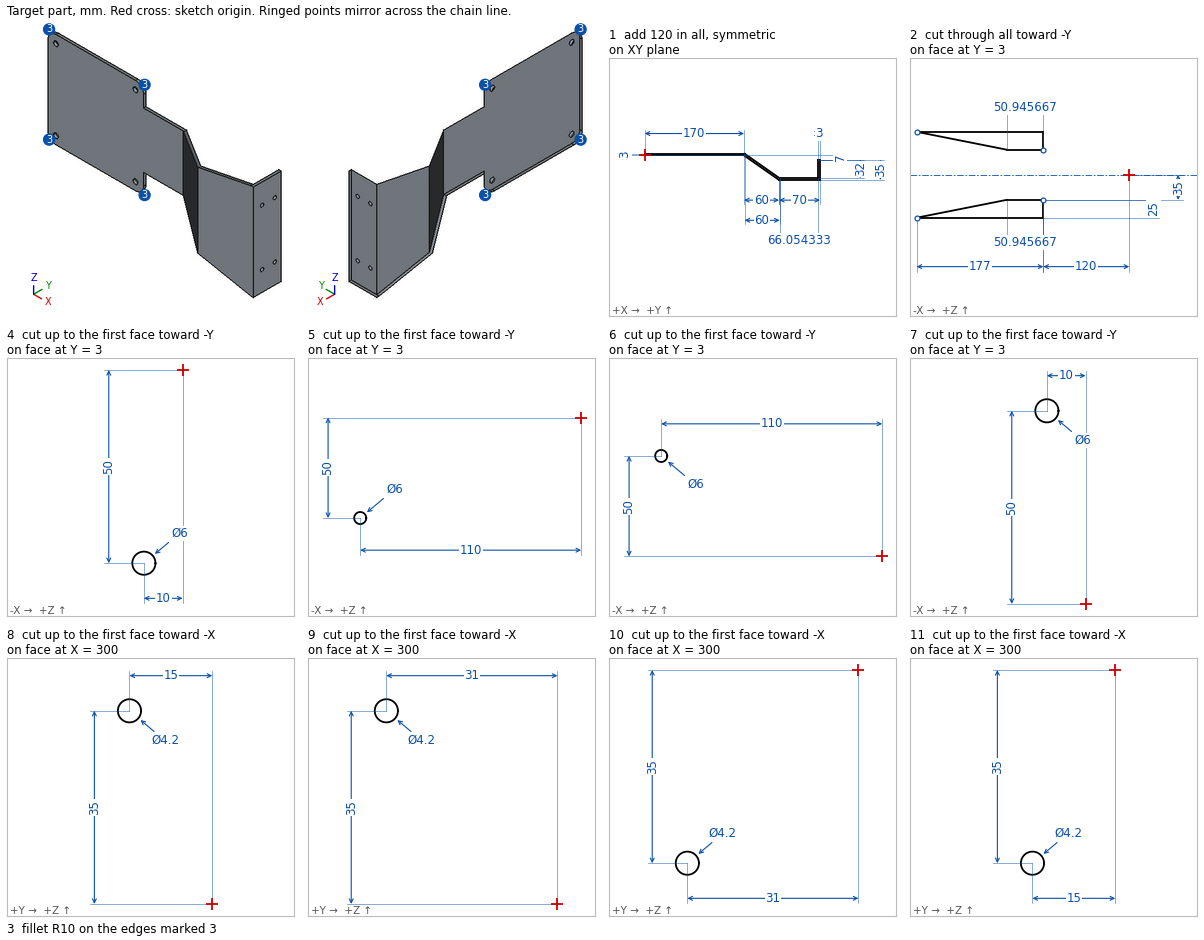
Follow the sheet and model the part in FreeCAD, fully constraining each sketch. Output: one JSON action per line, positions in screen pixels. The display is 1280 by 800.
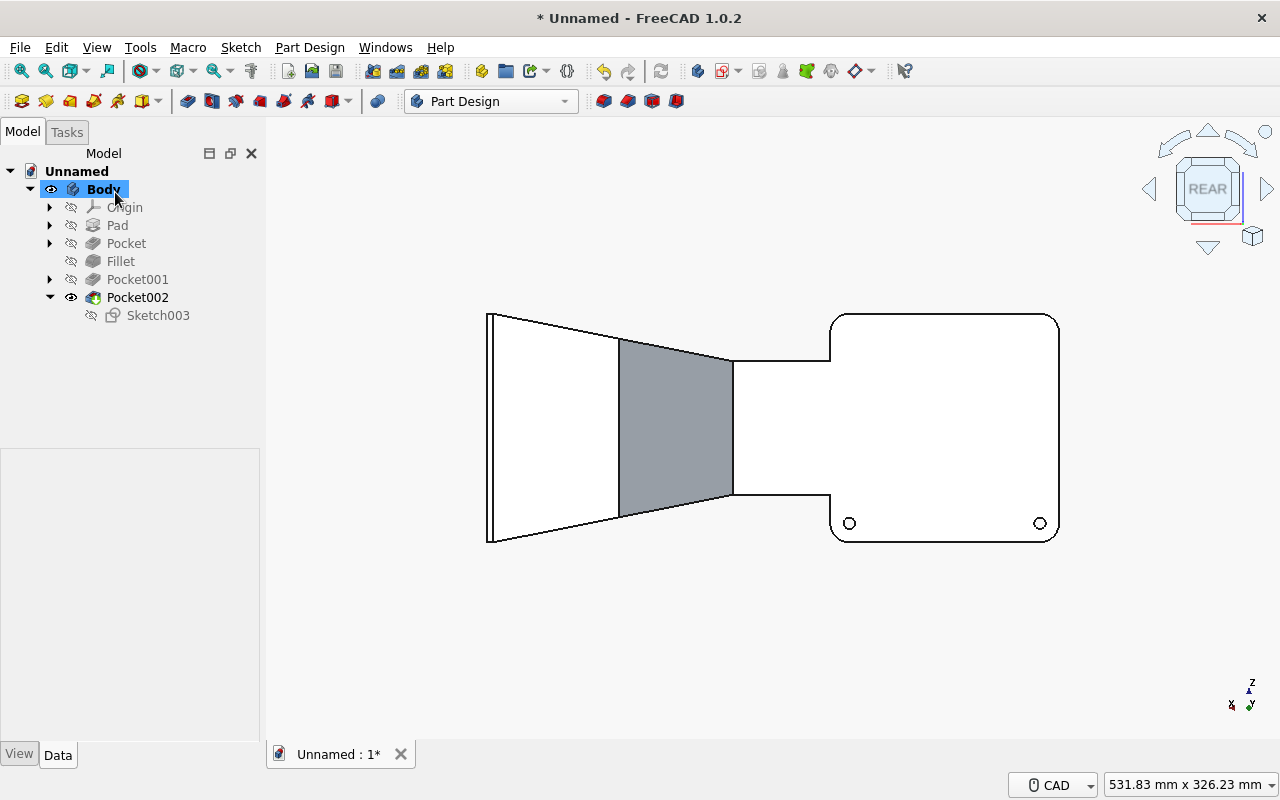
{"action": "left_click", "coordinate": [943, 427]}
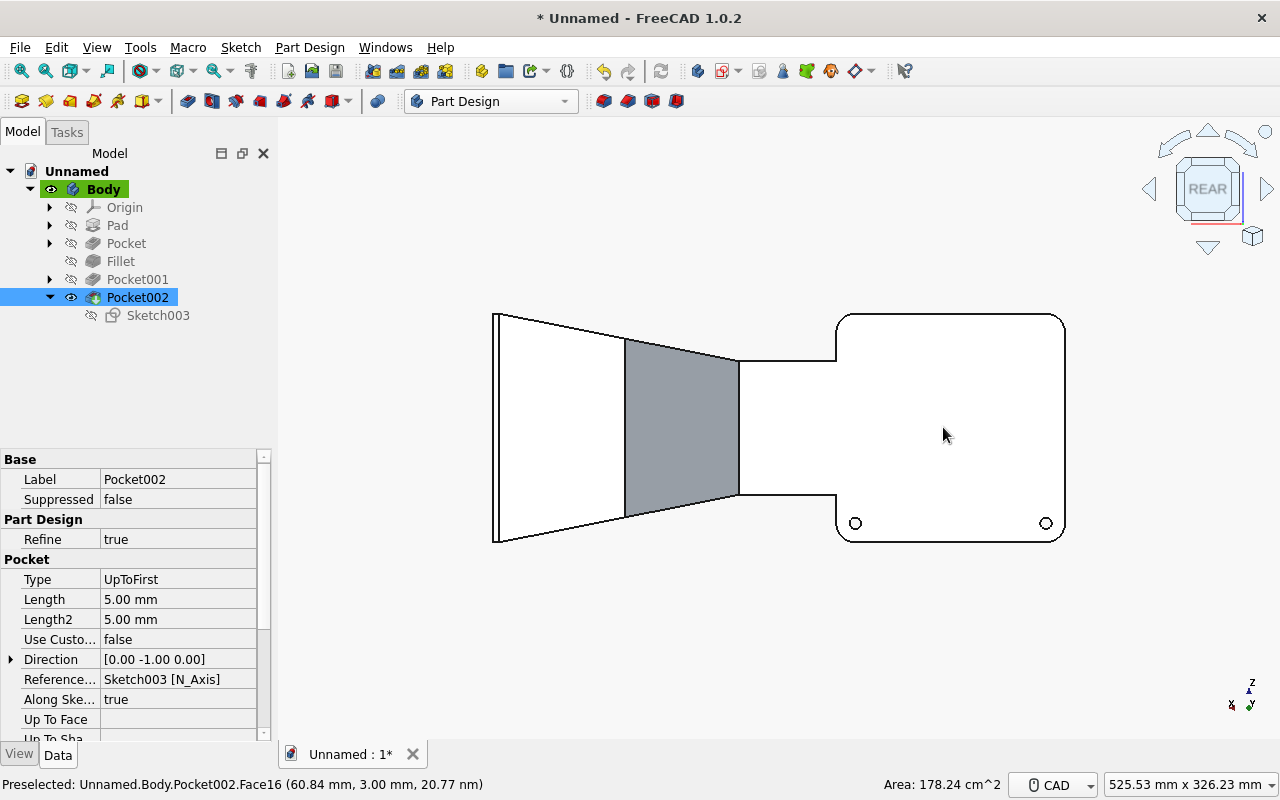
{"action": "left_click", "coordinate": [722, 72]}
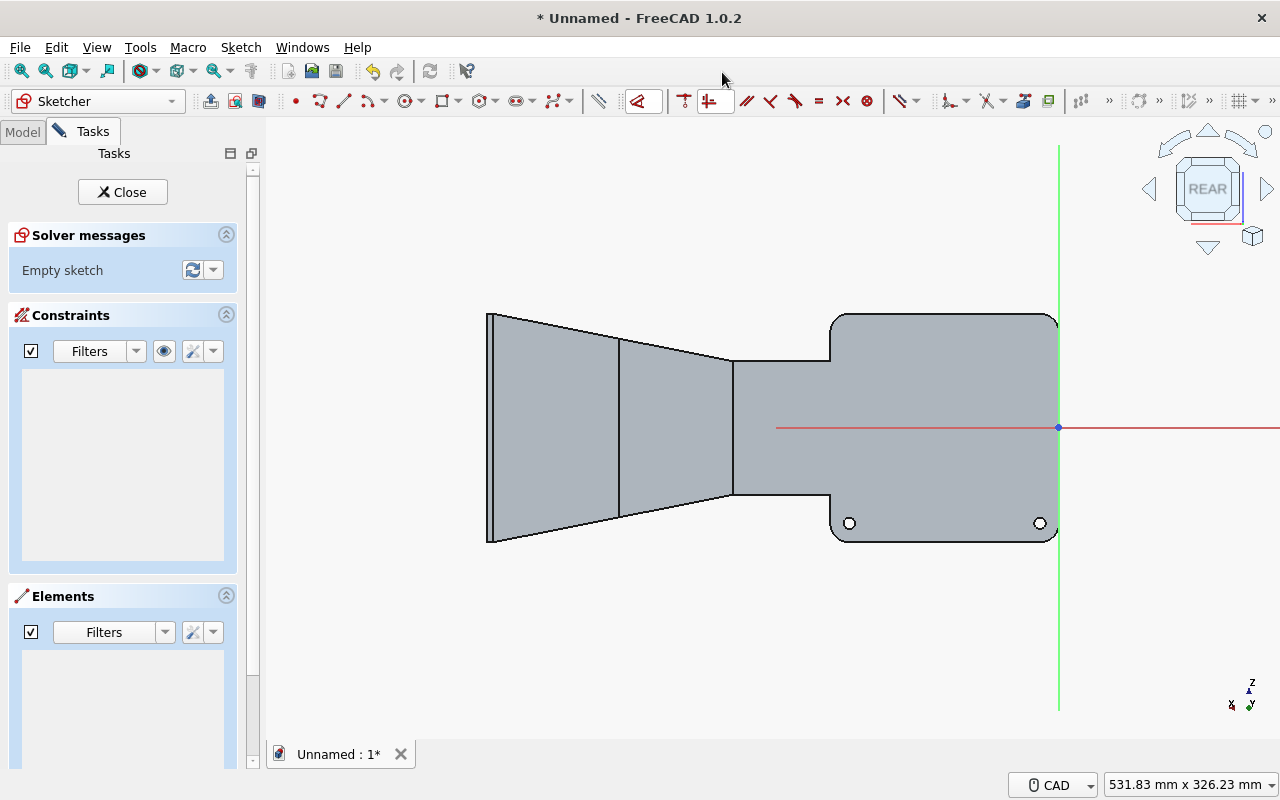
{"action": "scroll", "coordinate": [857, 328], "scroll_direction": "up", "scroll_amount": 15}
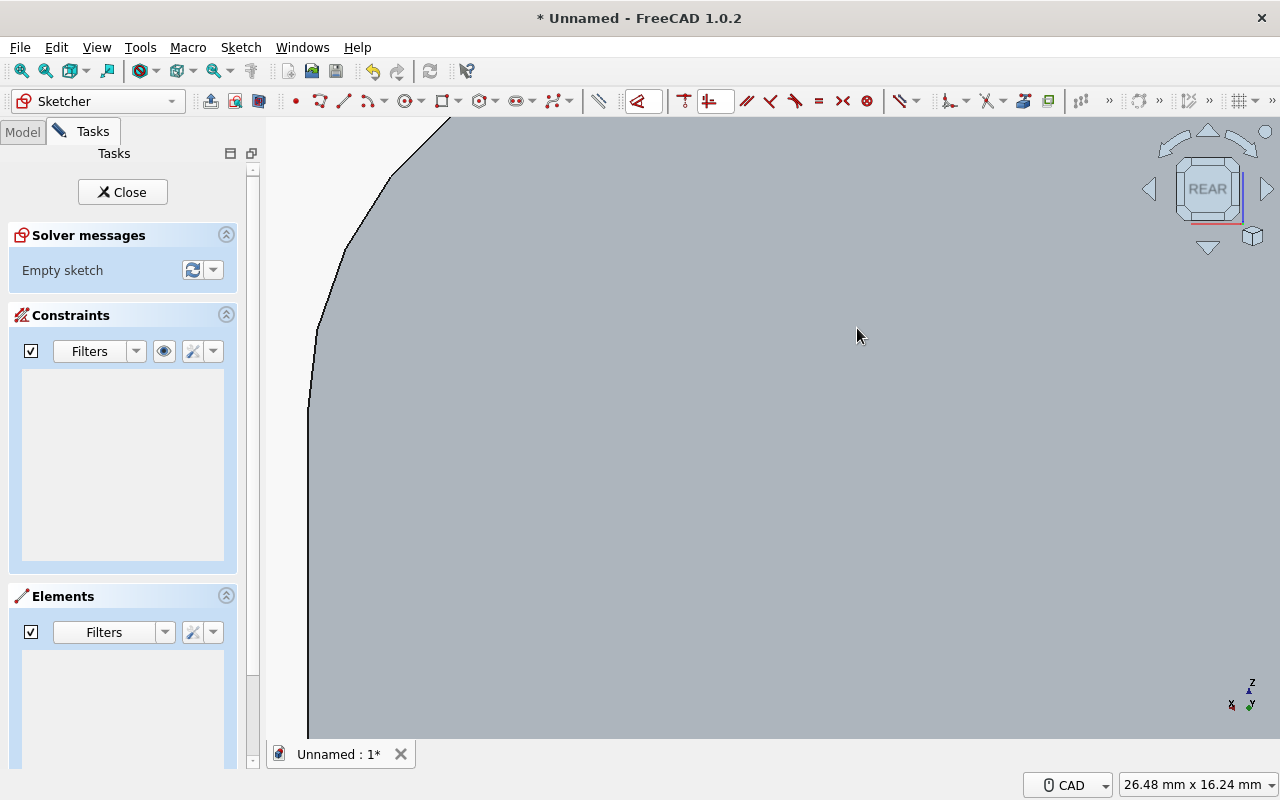
{"action": "scroll", "coordinate": [674, 400], "scroll_direction": "up", "scroll_amount": 3}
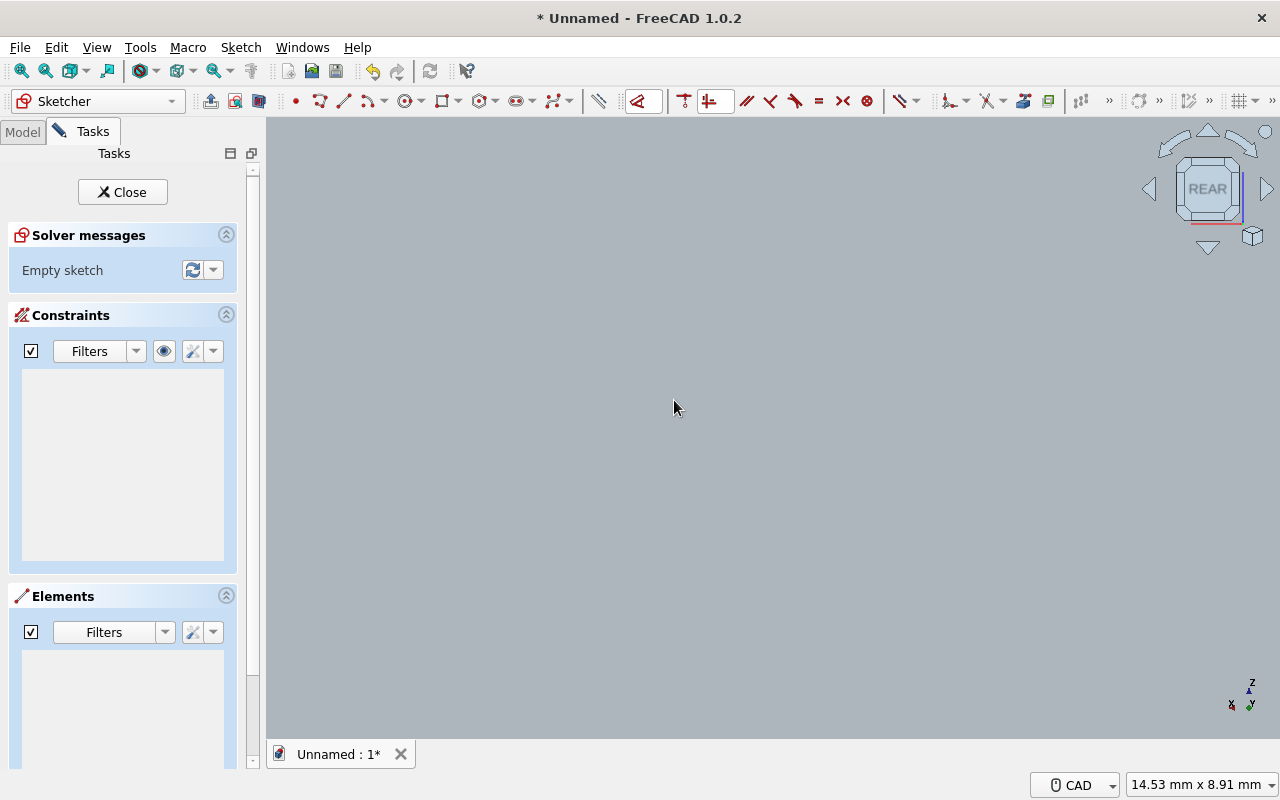
{"action": "left_click", "coordinate": [406, 102]}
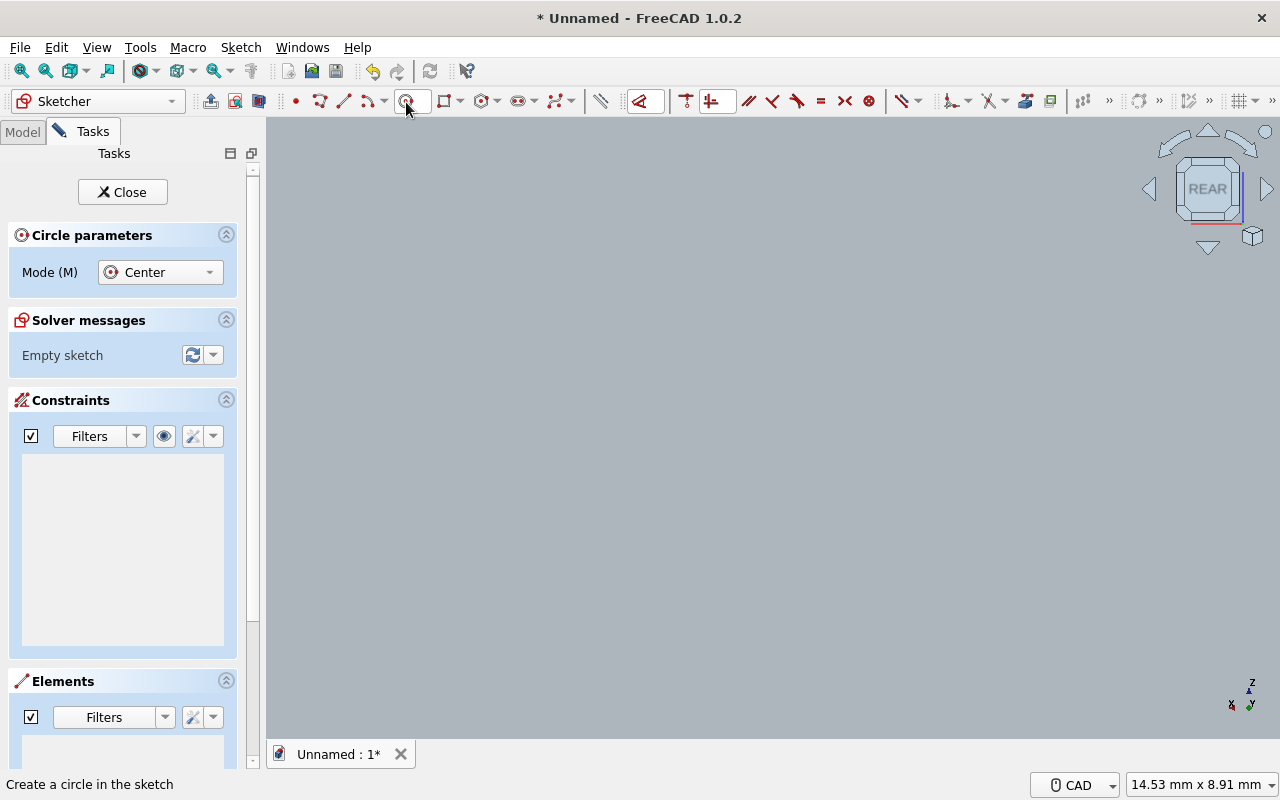
{"action": "left_click", "coordinate": [704, 427]}
{"action": "left_click", "coordinate": [852, 279]}
{"action": "key", "text": "Escape"}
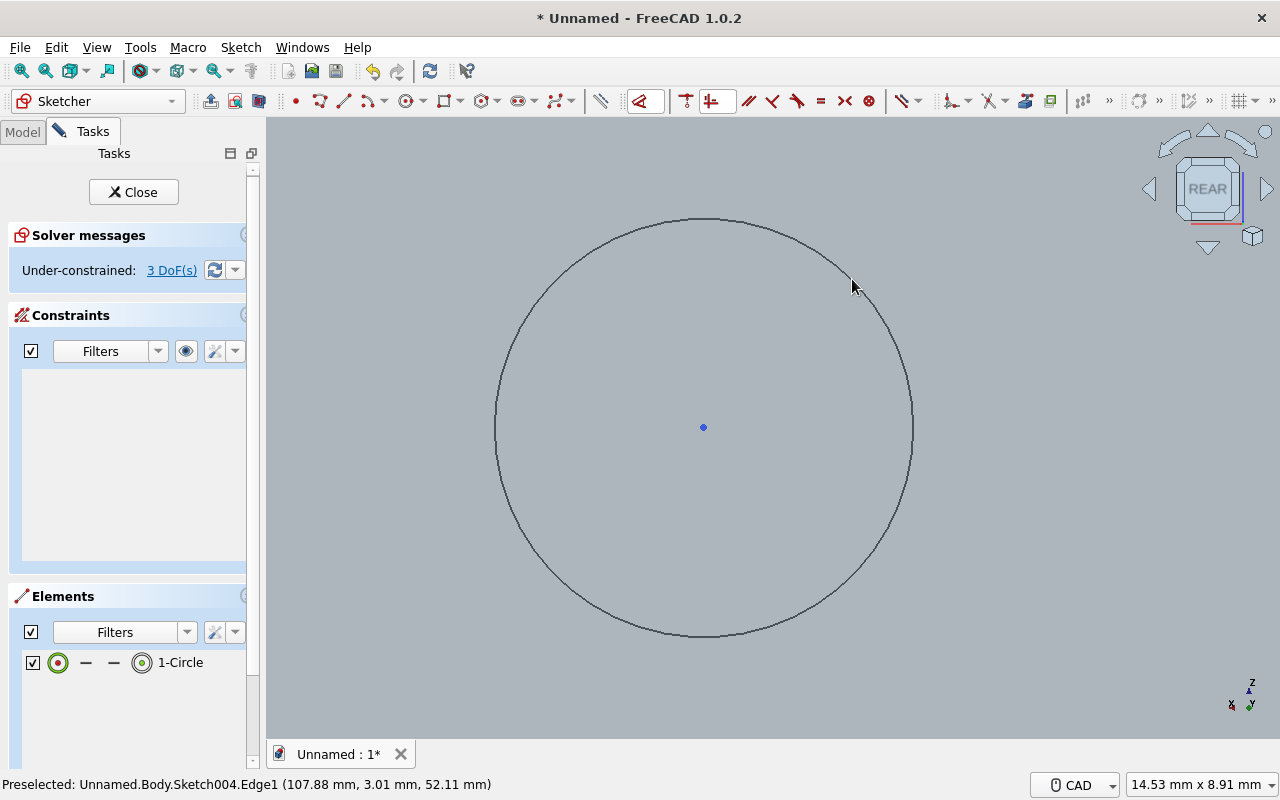
{"action": "left_click", "coordinate": [852, 280]}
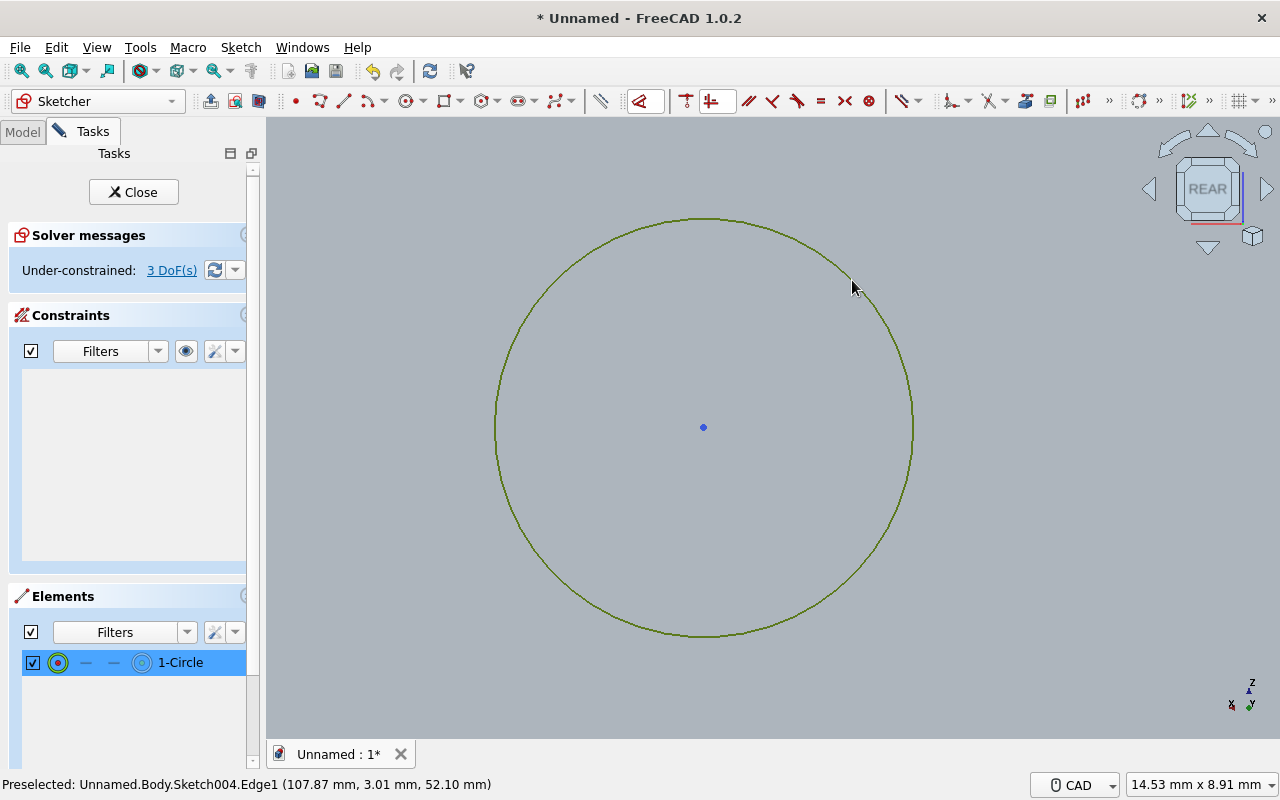
{"action": "key", "text": "k o"}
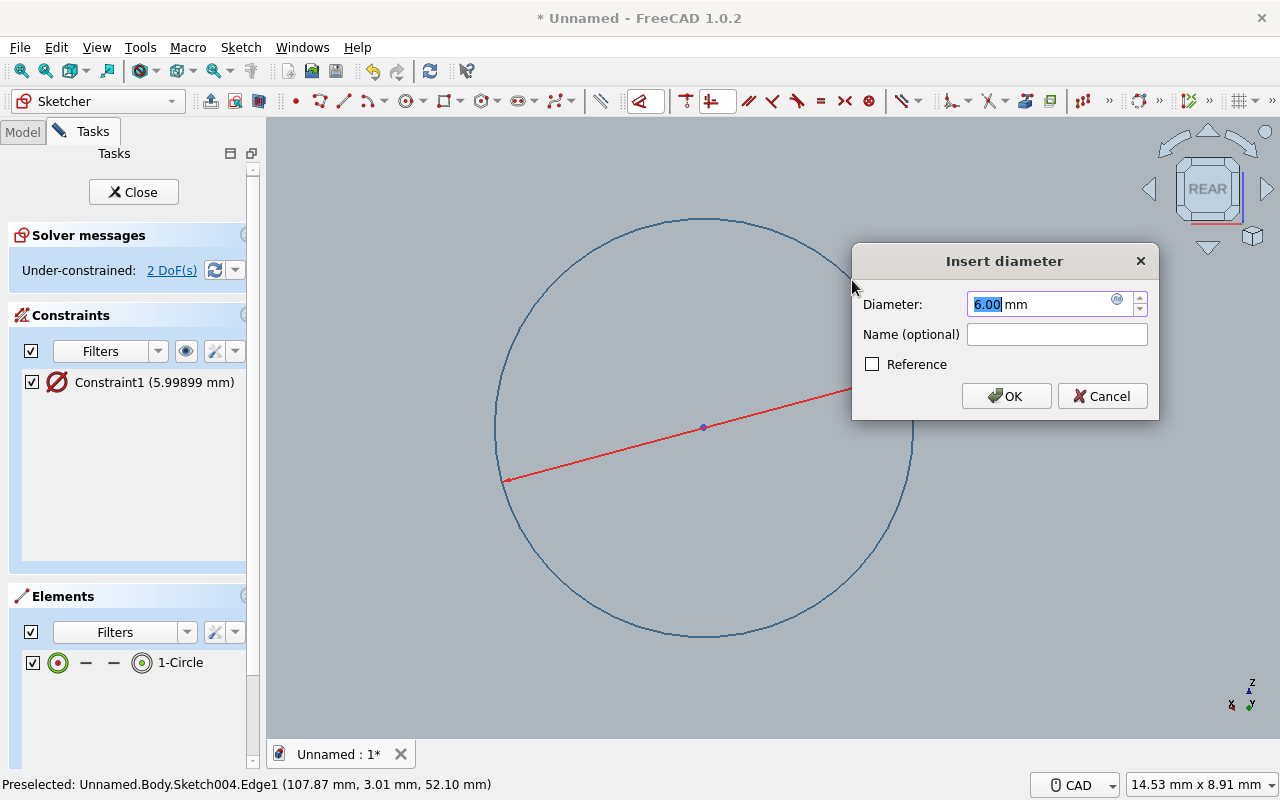
{"action": "type", "text": "6"}
{"action": "key", "text": "Return"}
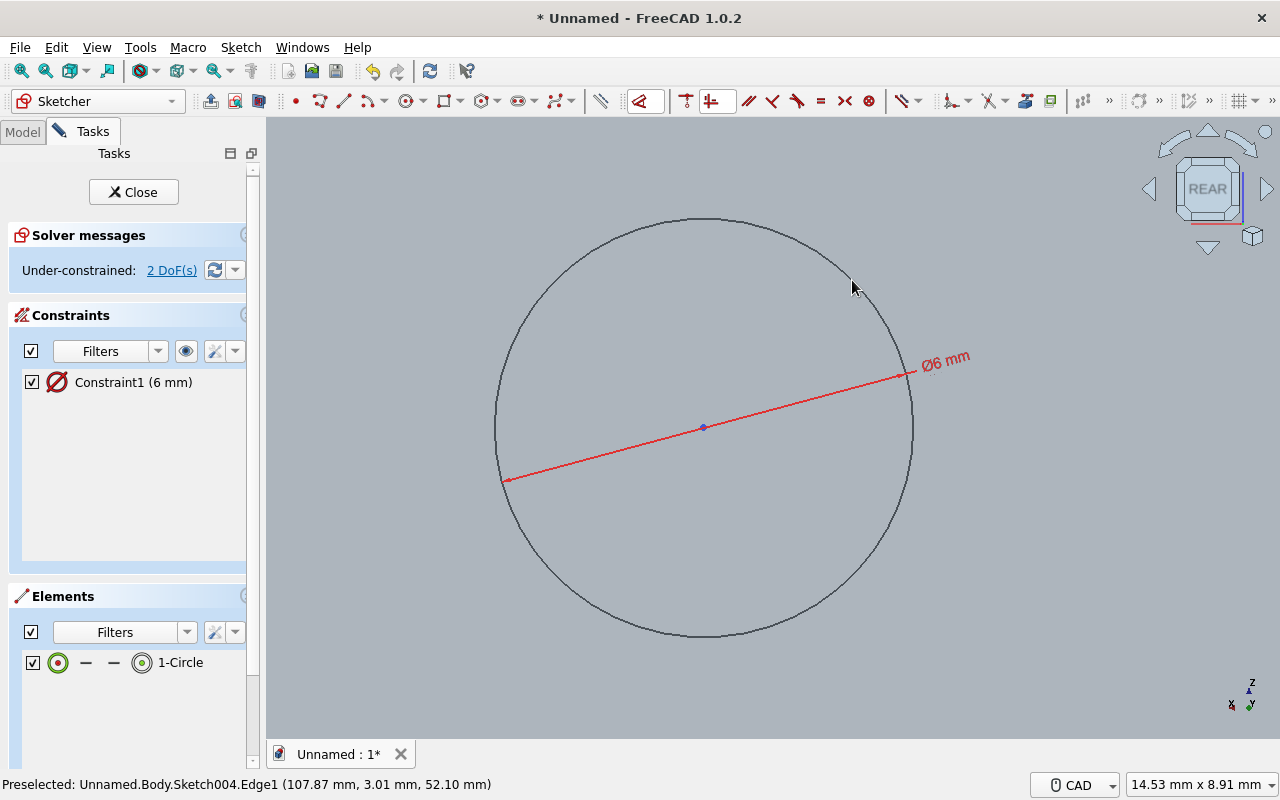
{"action": "left_click", "coordinate": [704, 428]}